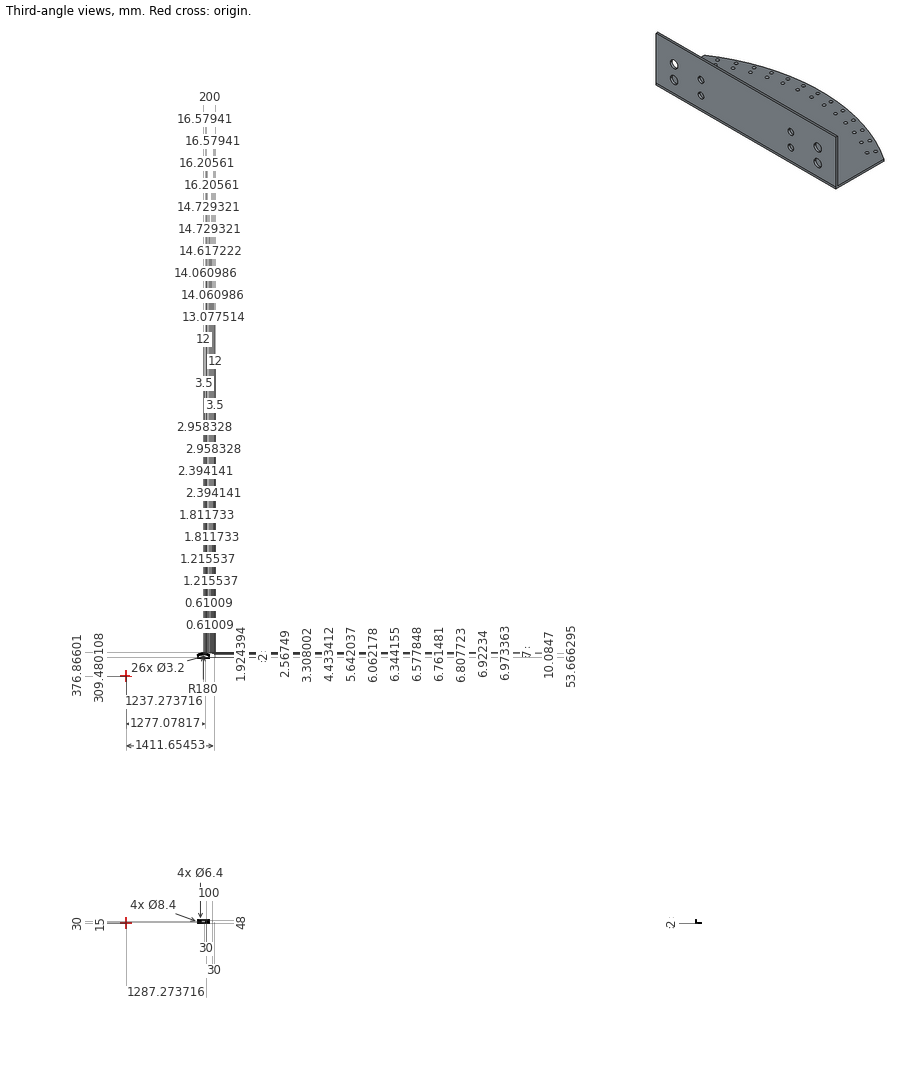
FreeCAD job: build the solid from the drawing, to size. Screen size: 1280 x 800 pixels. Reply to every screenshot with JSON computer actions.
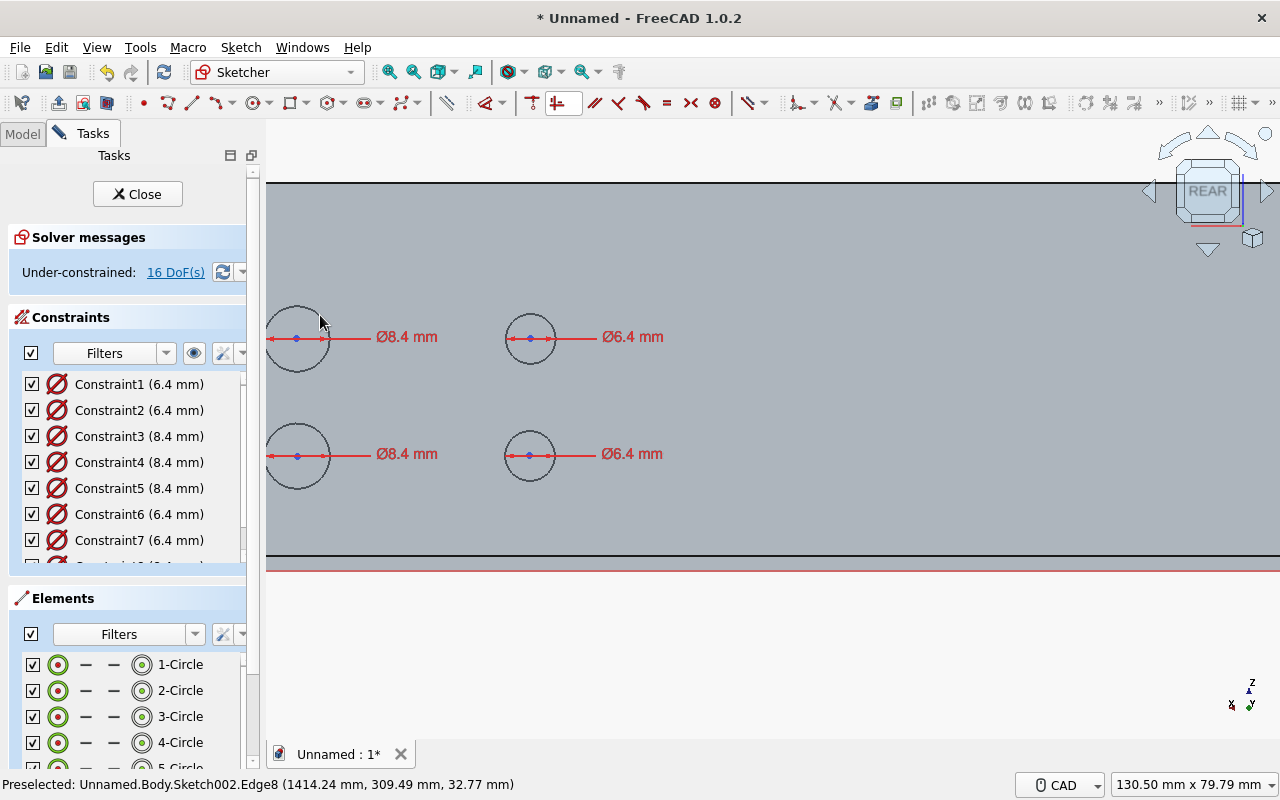
{"action": "scroll", "coordinate": [530, 456], "scroll_direction": "down", "scroll_amount": 4}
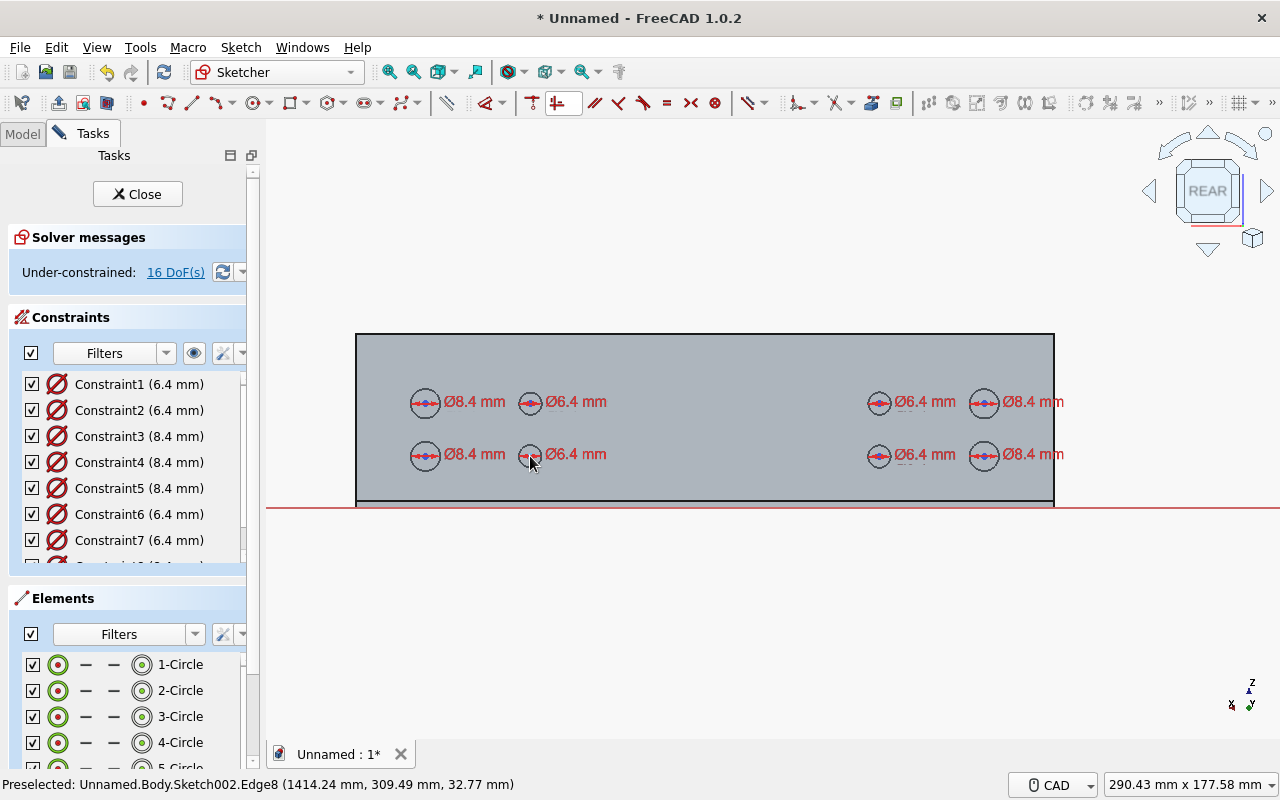
{"action": "left_click", "coordinate": [880, 404]}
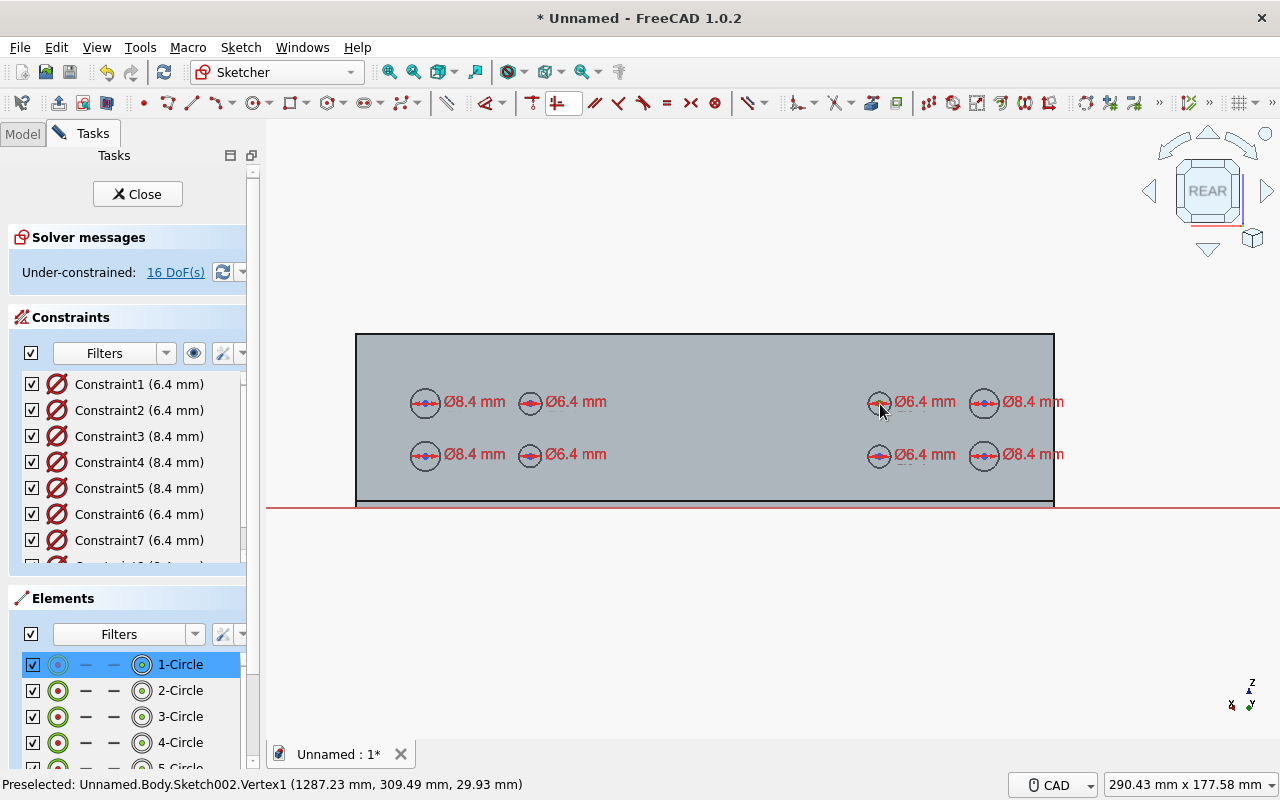
{"action": "left_click", "coordinate": [530, 404]}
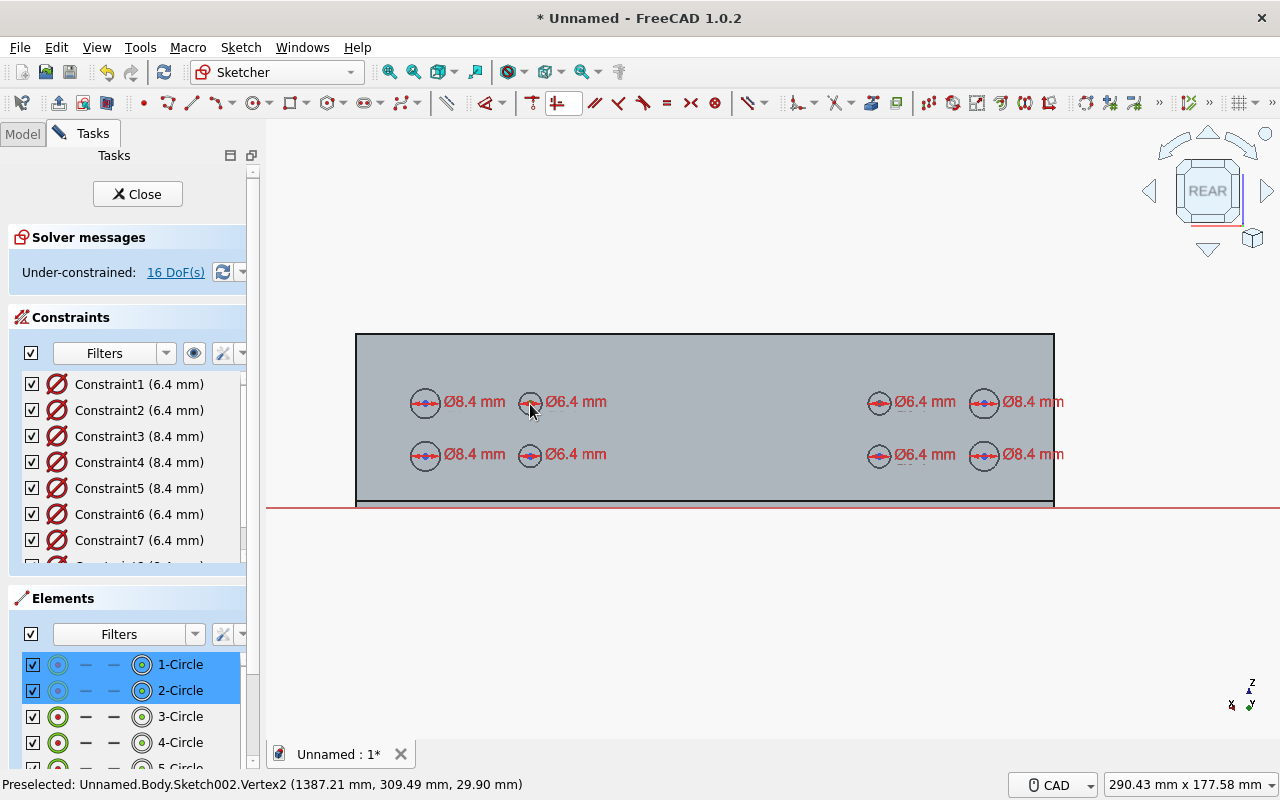
{"action": "key", "text": "h"}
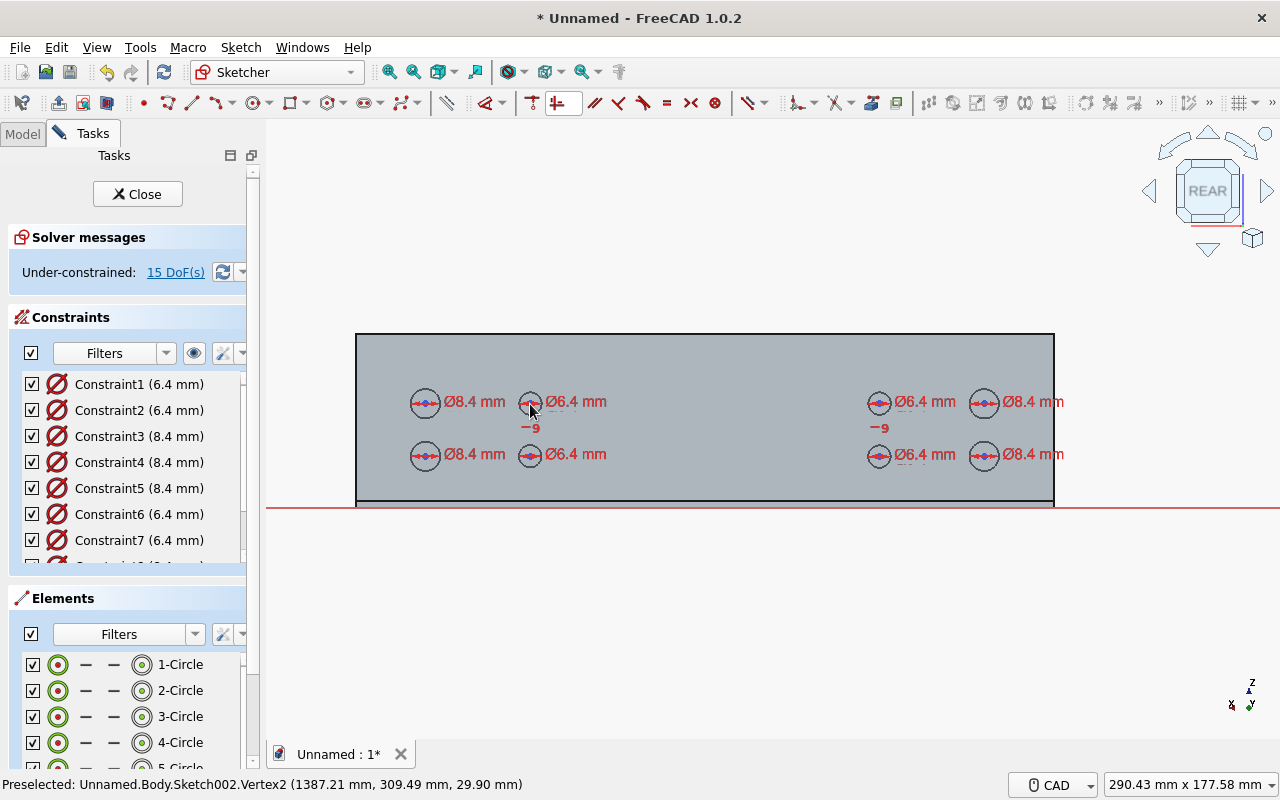
{"action": "left_click", "coordinate": [984, 456]}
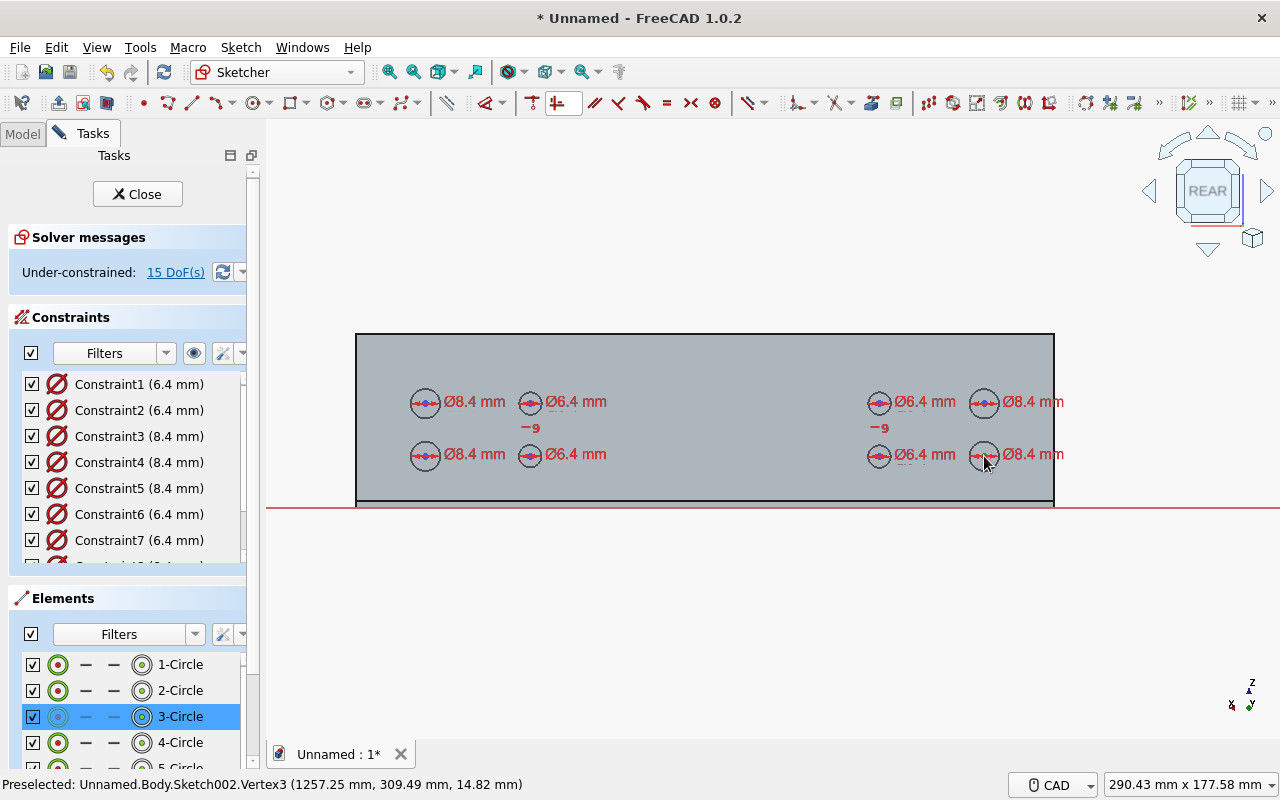
{"action": "left_click", "coordinate": [426, 456]}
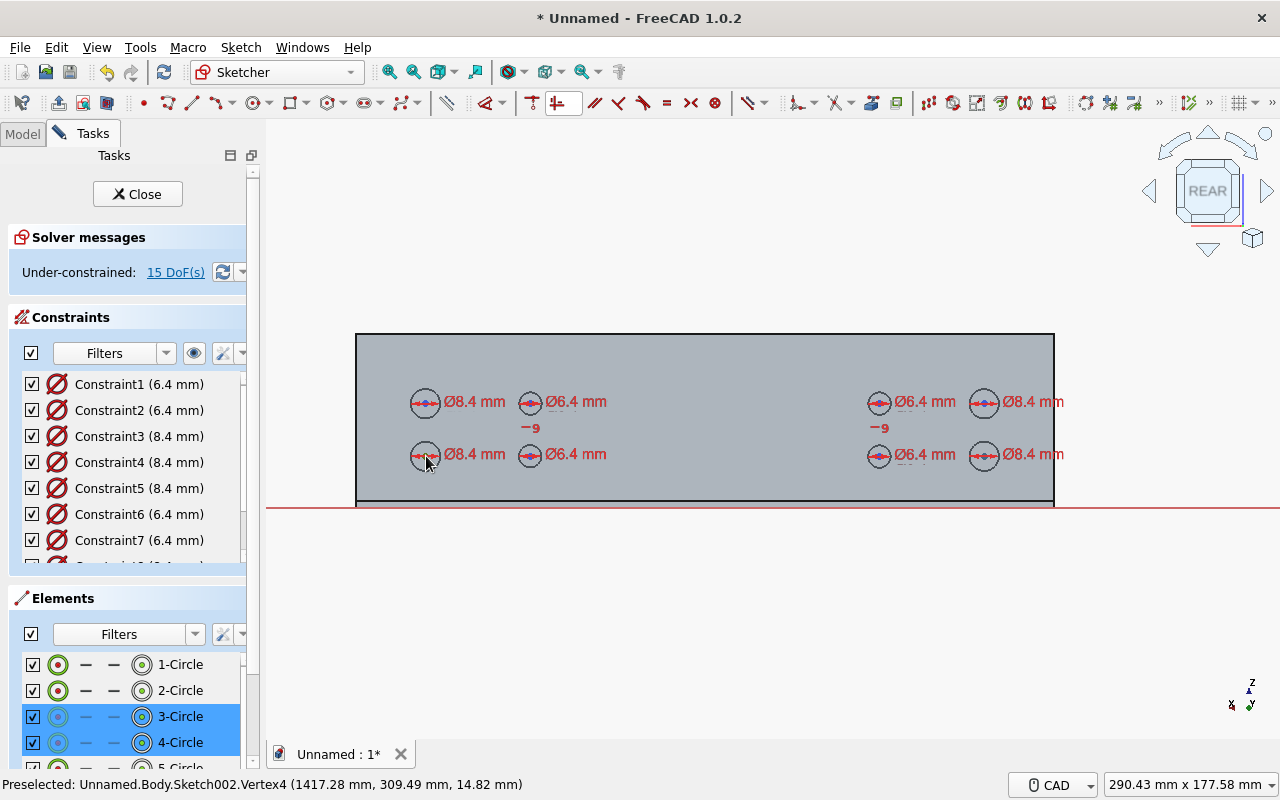
{"action": "key", "text": "h"}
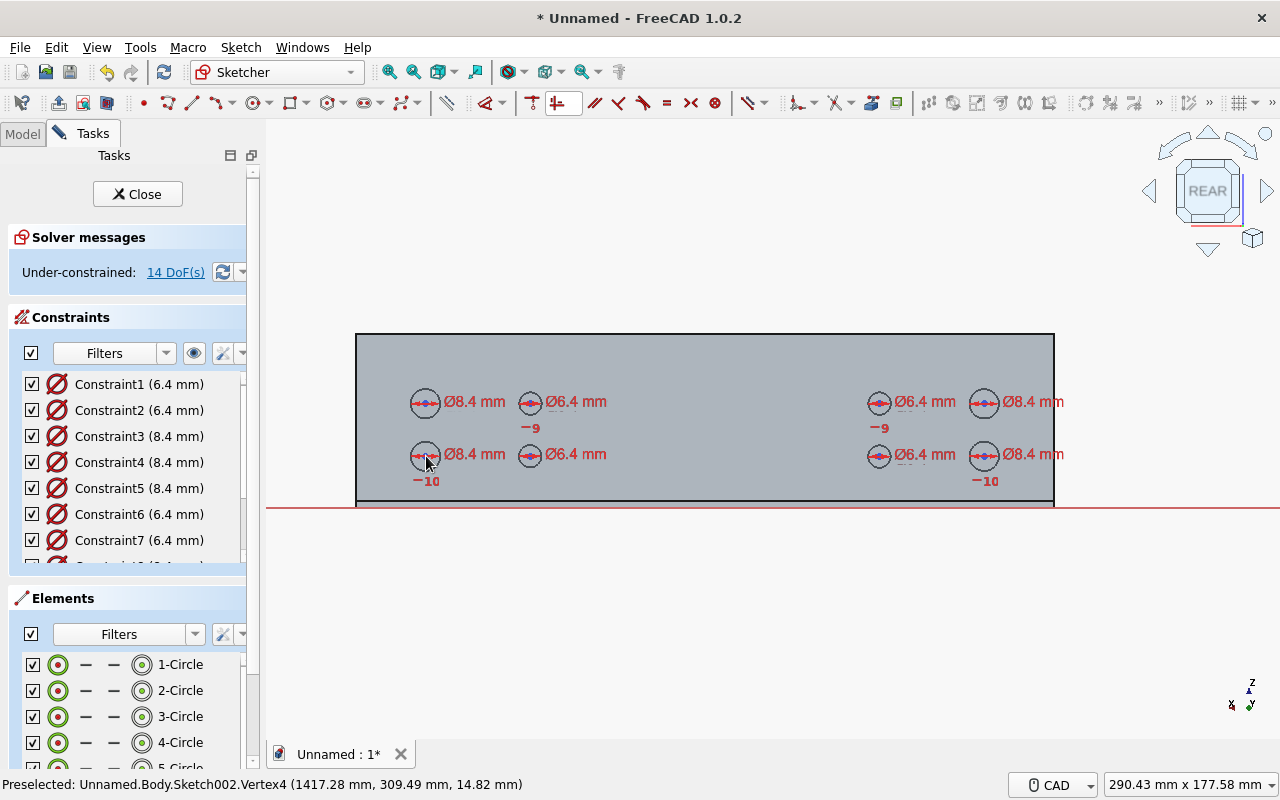
{"action": "left_click", "coordinate": [984, 456]}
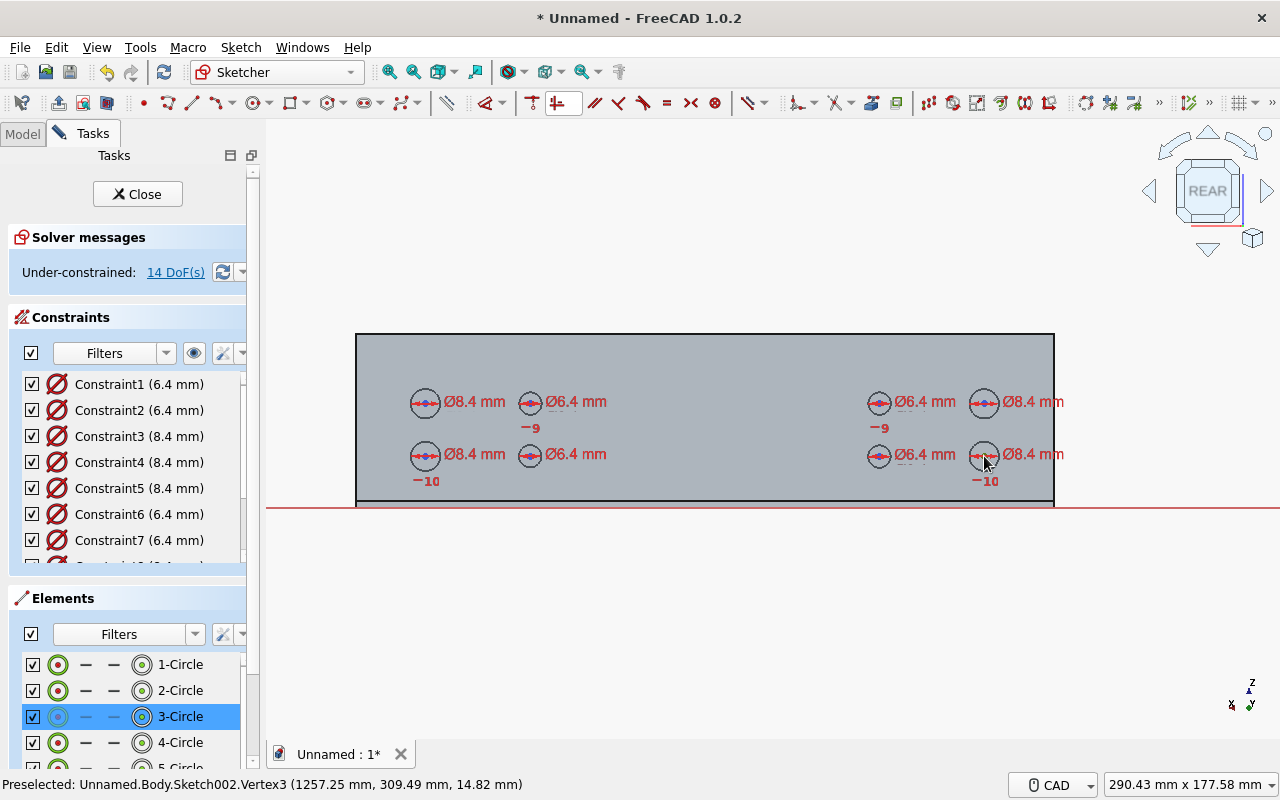
{"action": "left_click", "coordinate": [984, 404]}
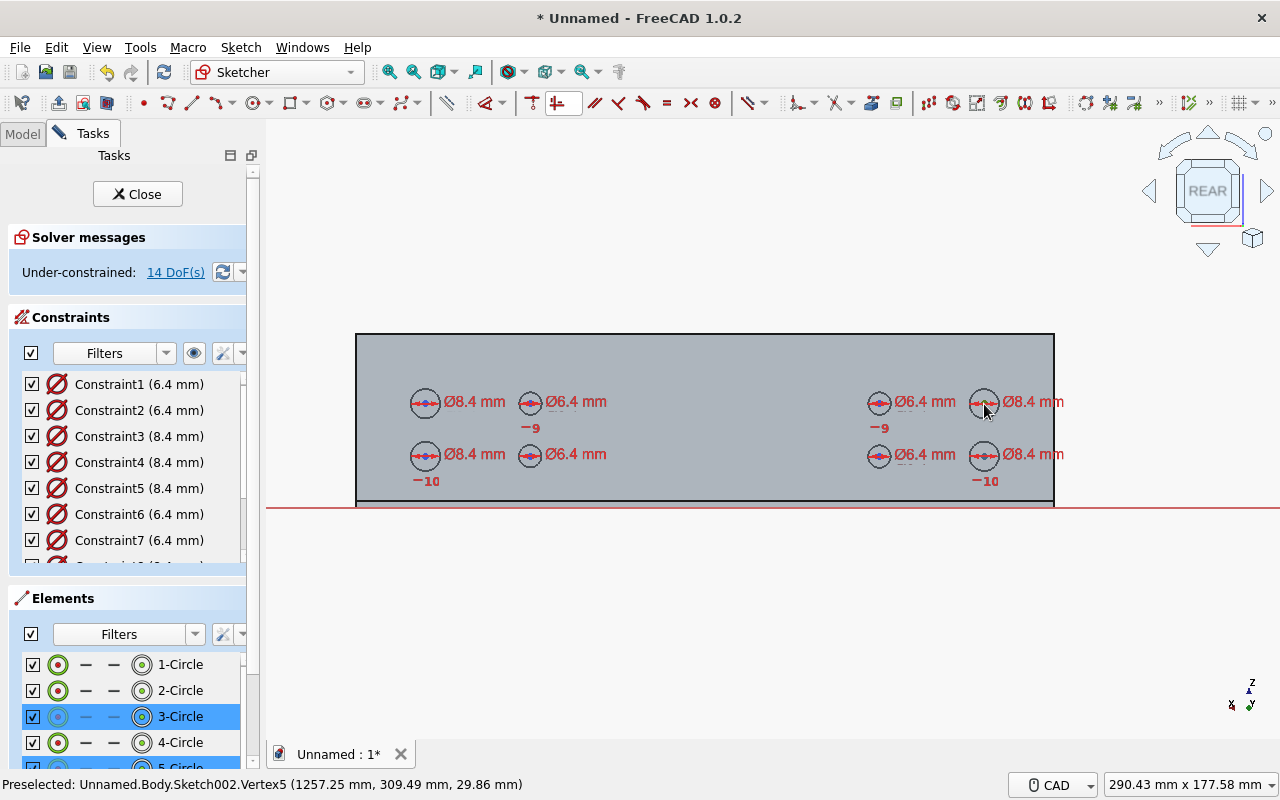
{"action": "key", "text": "v"}